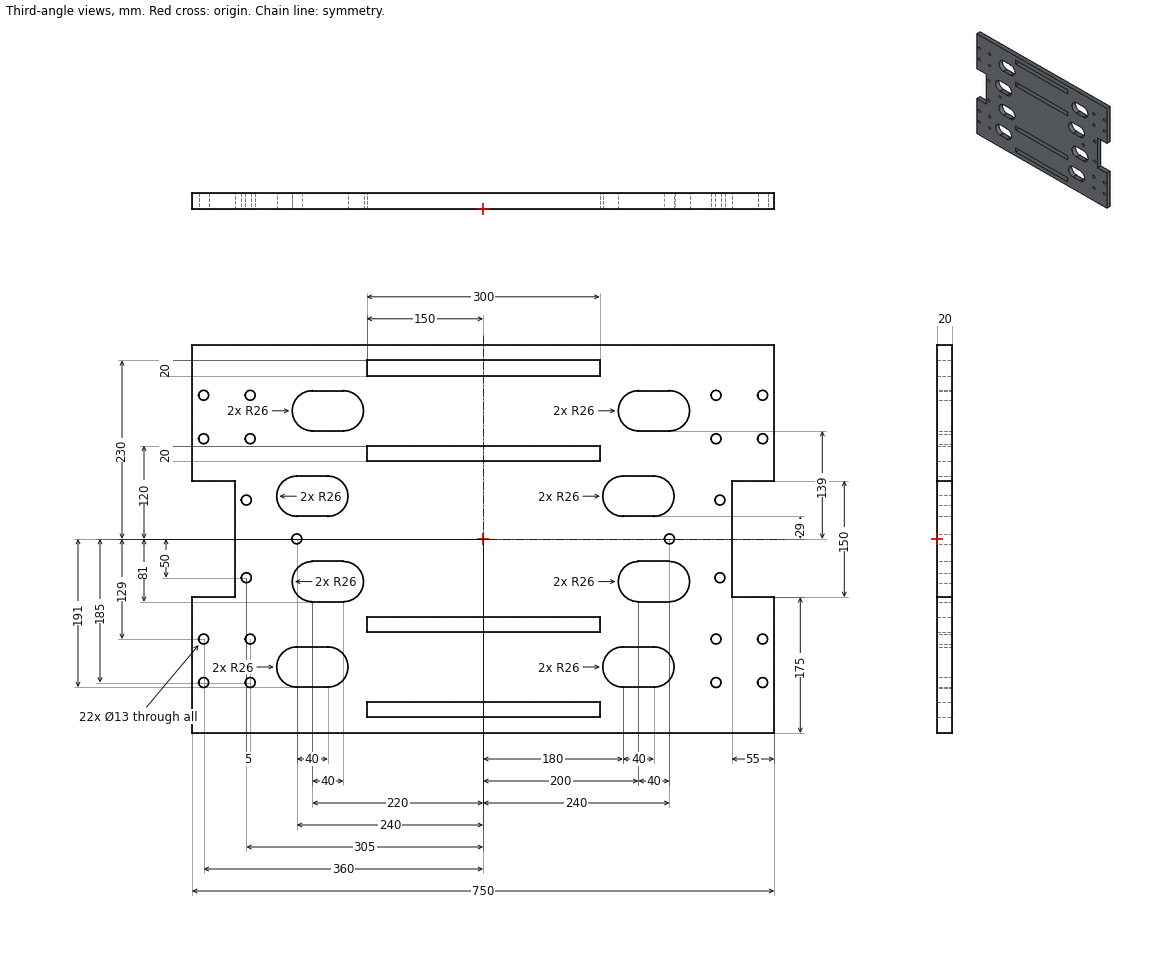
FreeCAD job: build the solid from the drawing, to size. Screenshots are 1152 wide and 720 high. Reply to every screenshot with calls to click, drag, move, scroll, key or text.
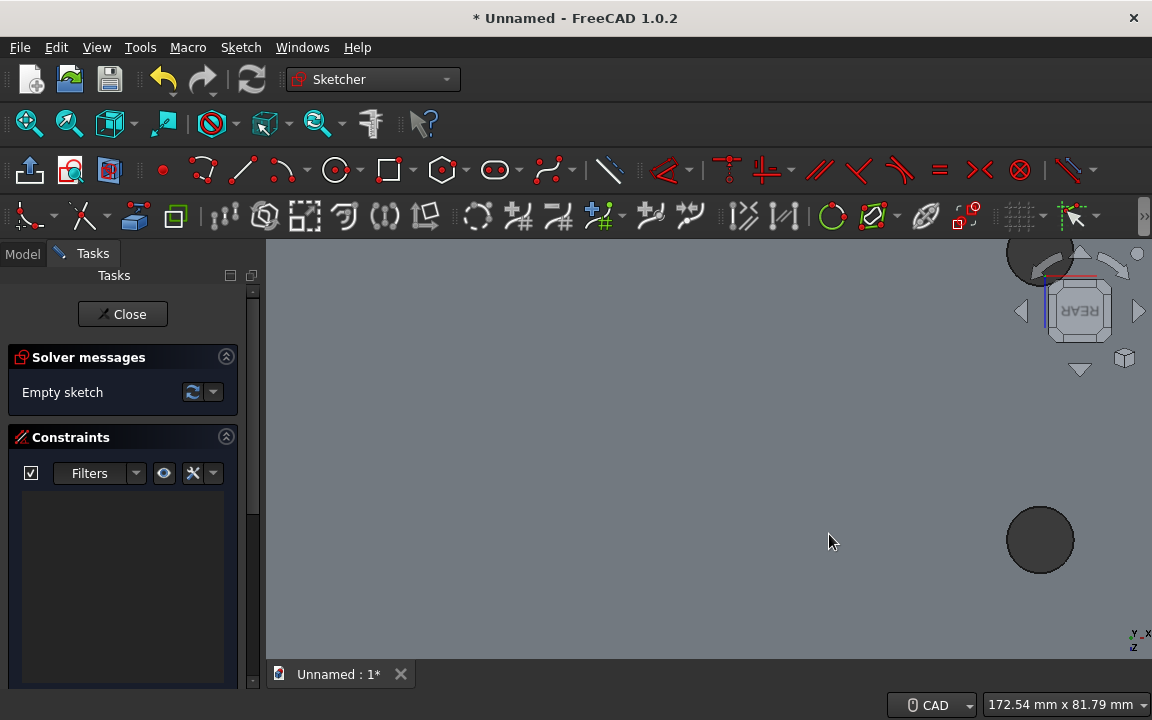
click(496, 170)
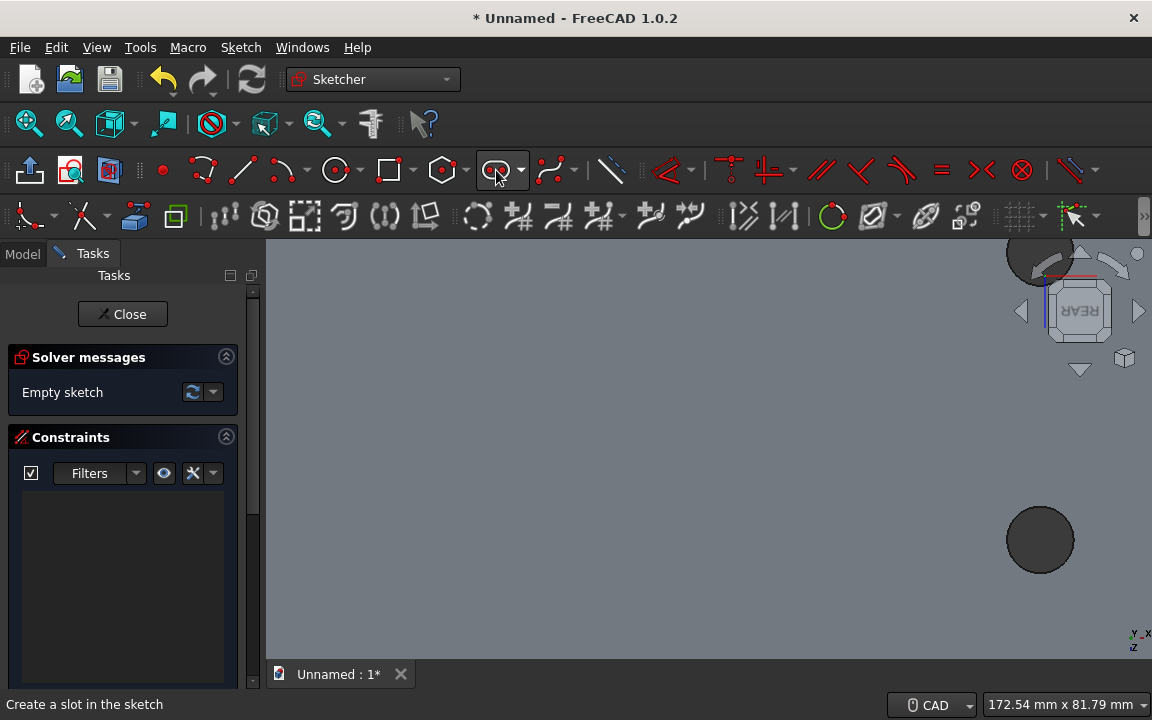
click(527, 437)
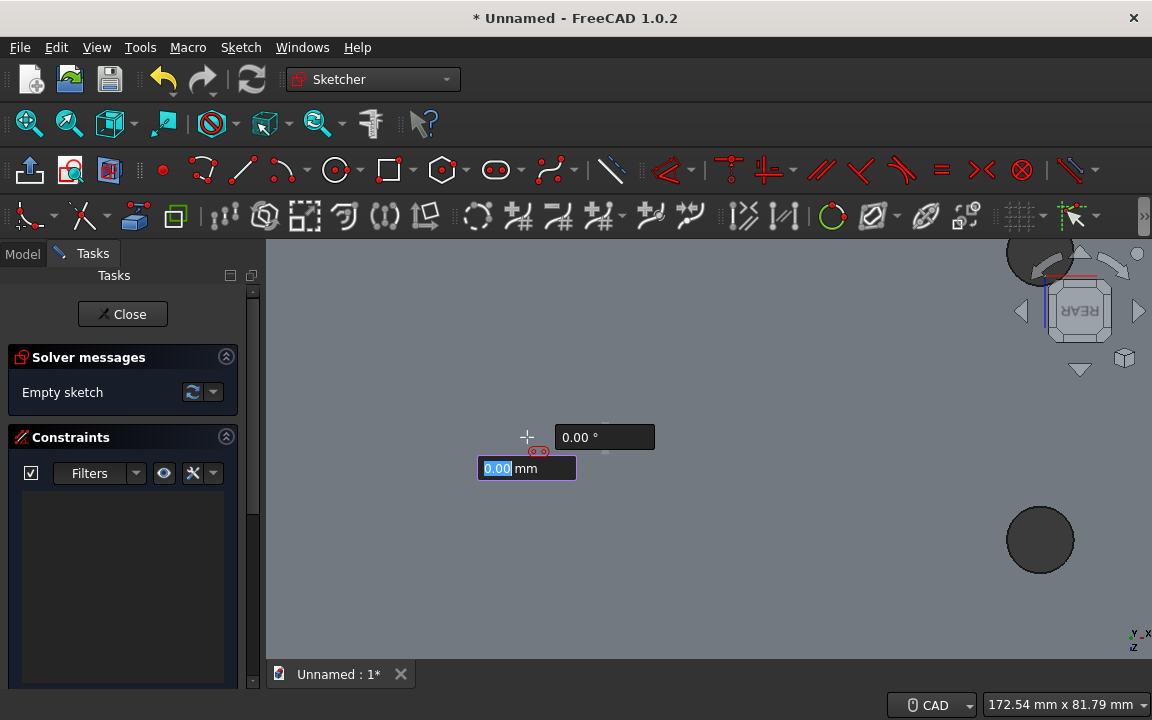
click(732, 437)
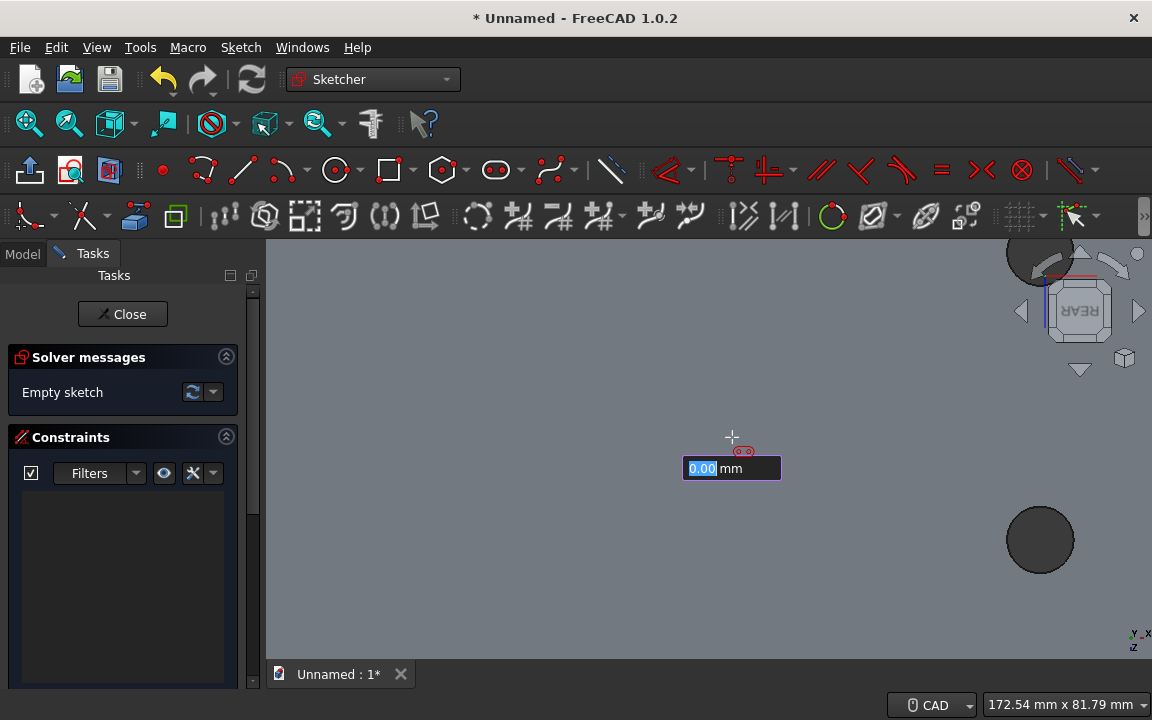
click(630, 304)
key(Escape)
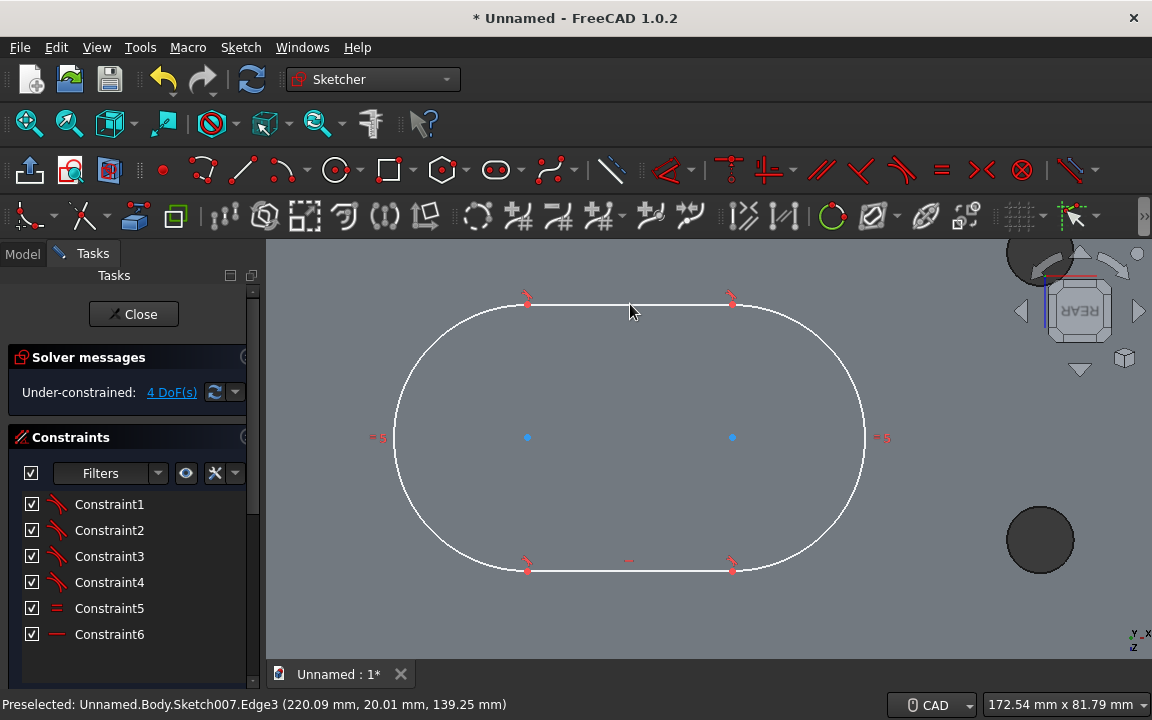
click(666, 170)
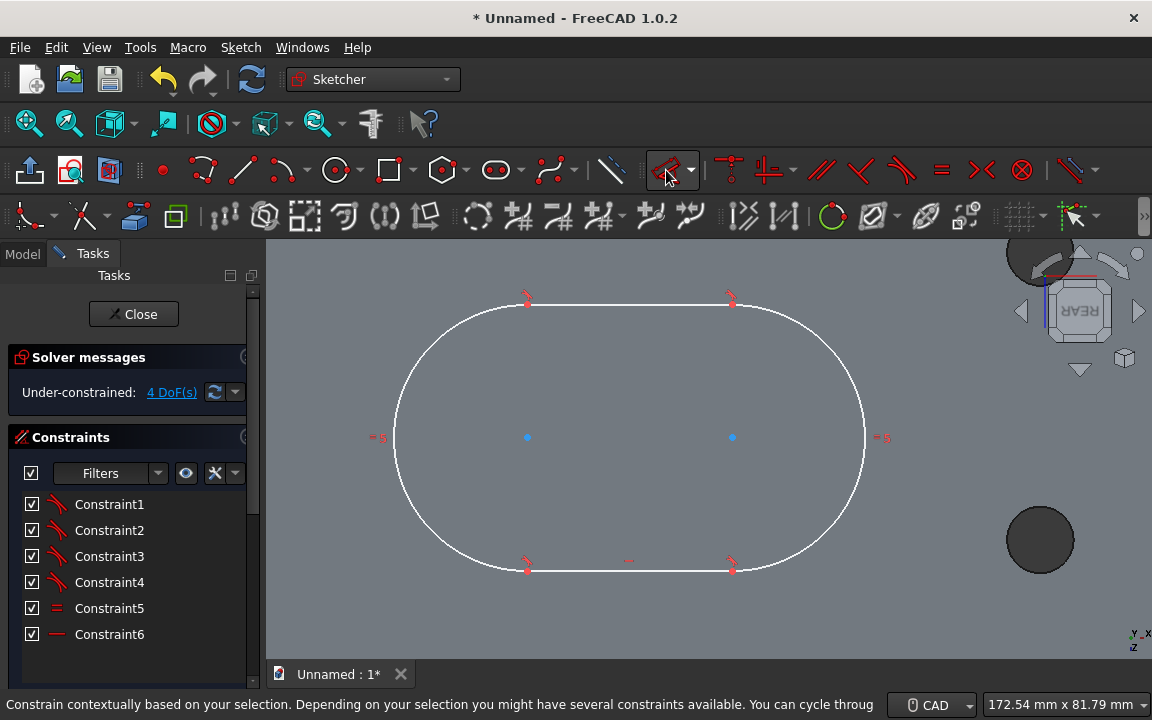
click(419, 360)
click(393, 341)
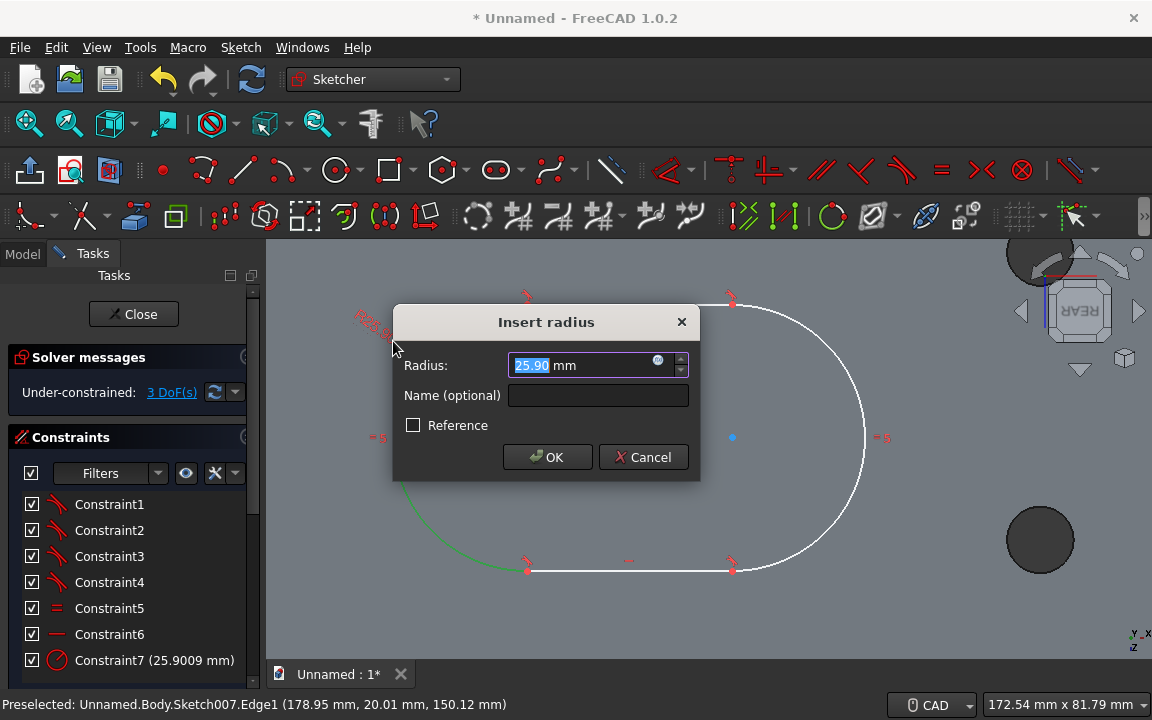
text(26)
key(Return)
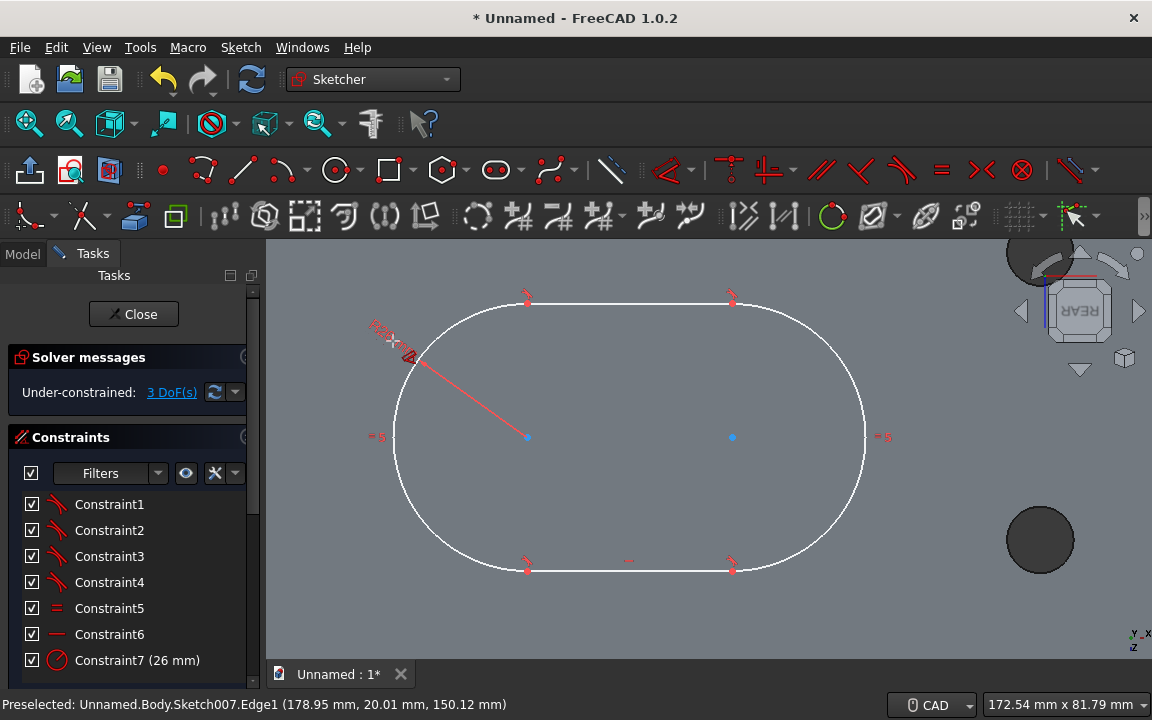
click(589, 304)
click(630, 270)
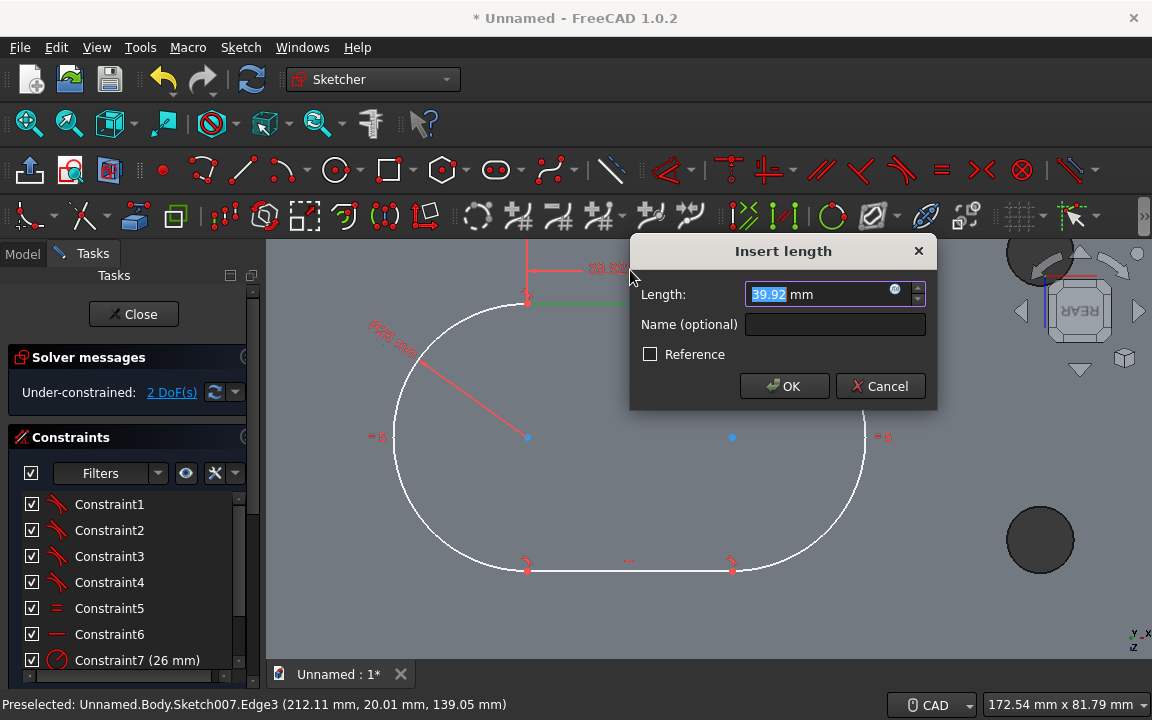
text(40)
key(Return)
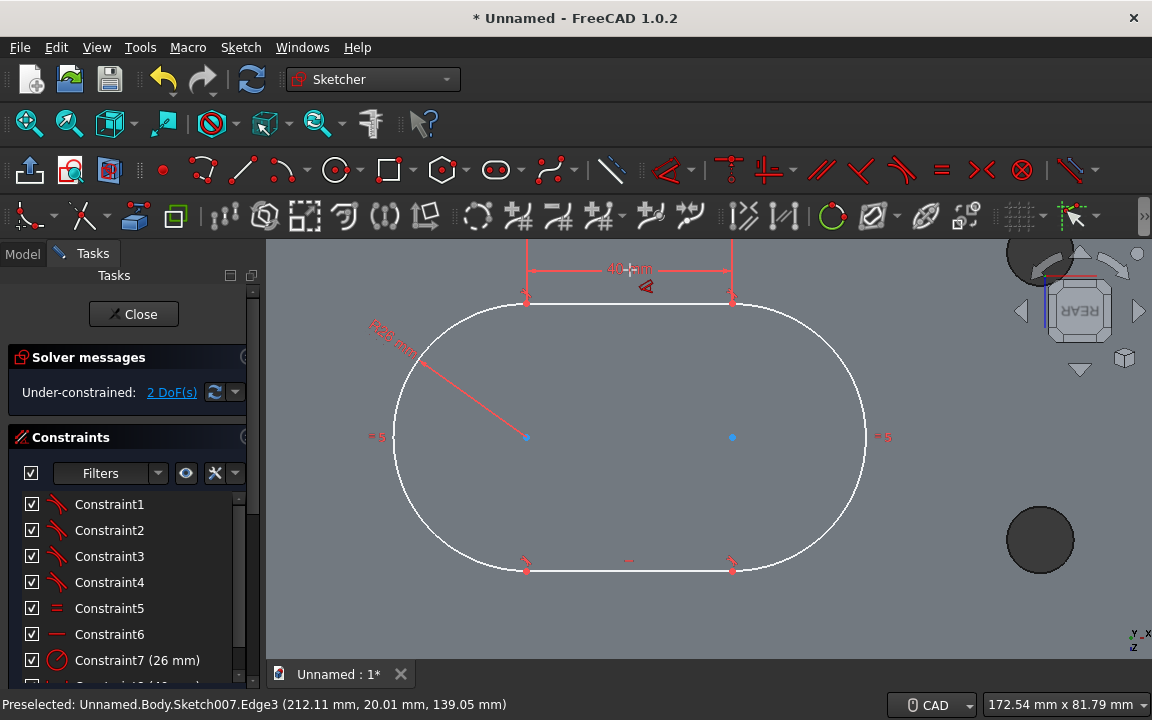
click(527, 304)
click(464, 338)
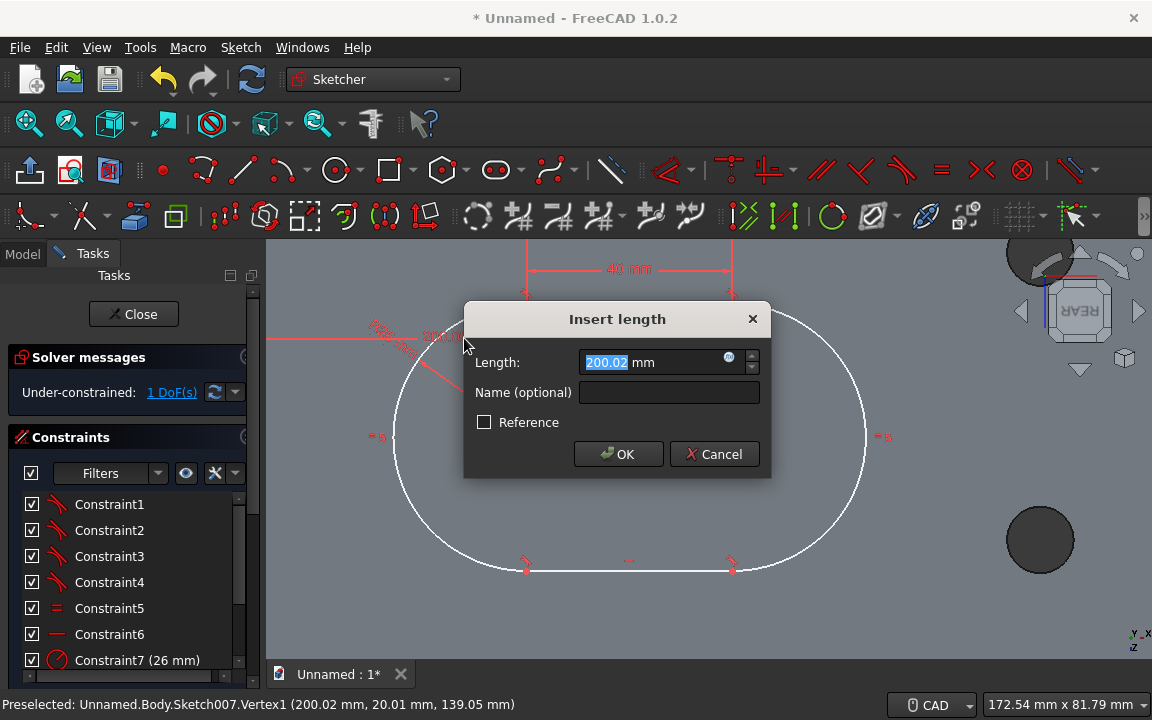
text(200)
key(Return)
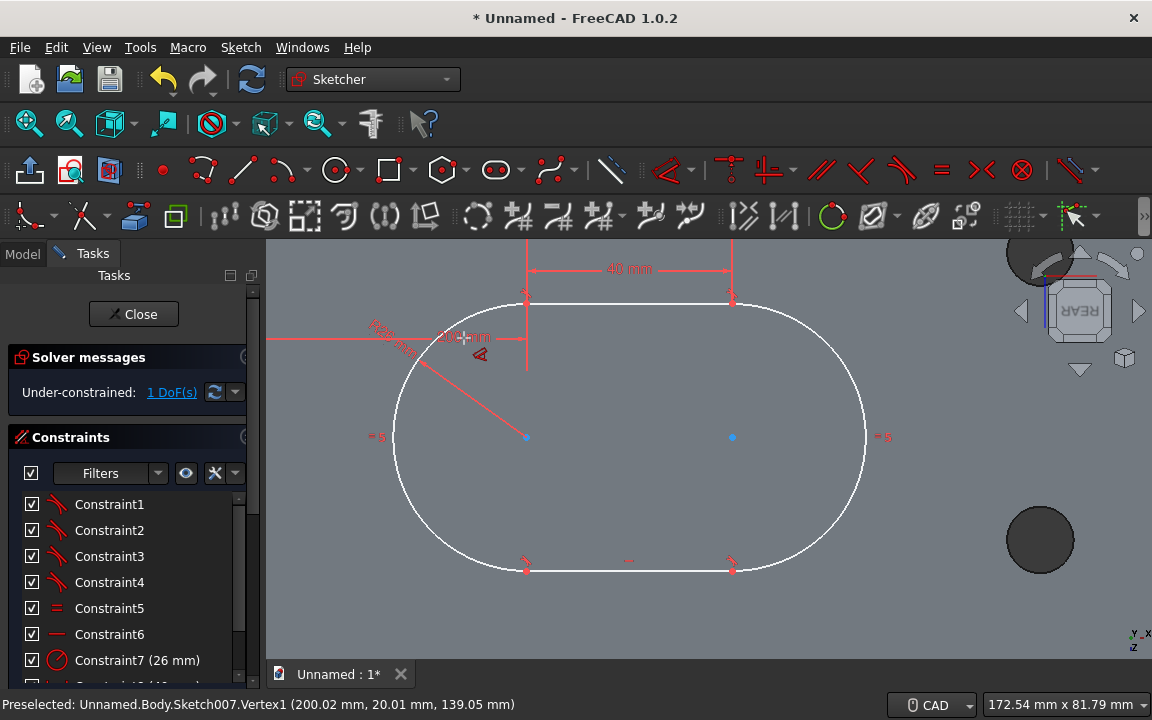
click(527, 304)
click(707, 285)